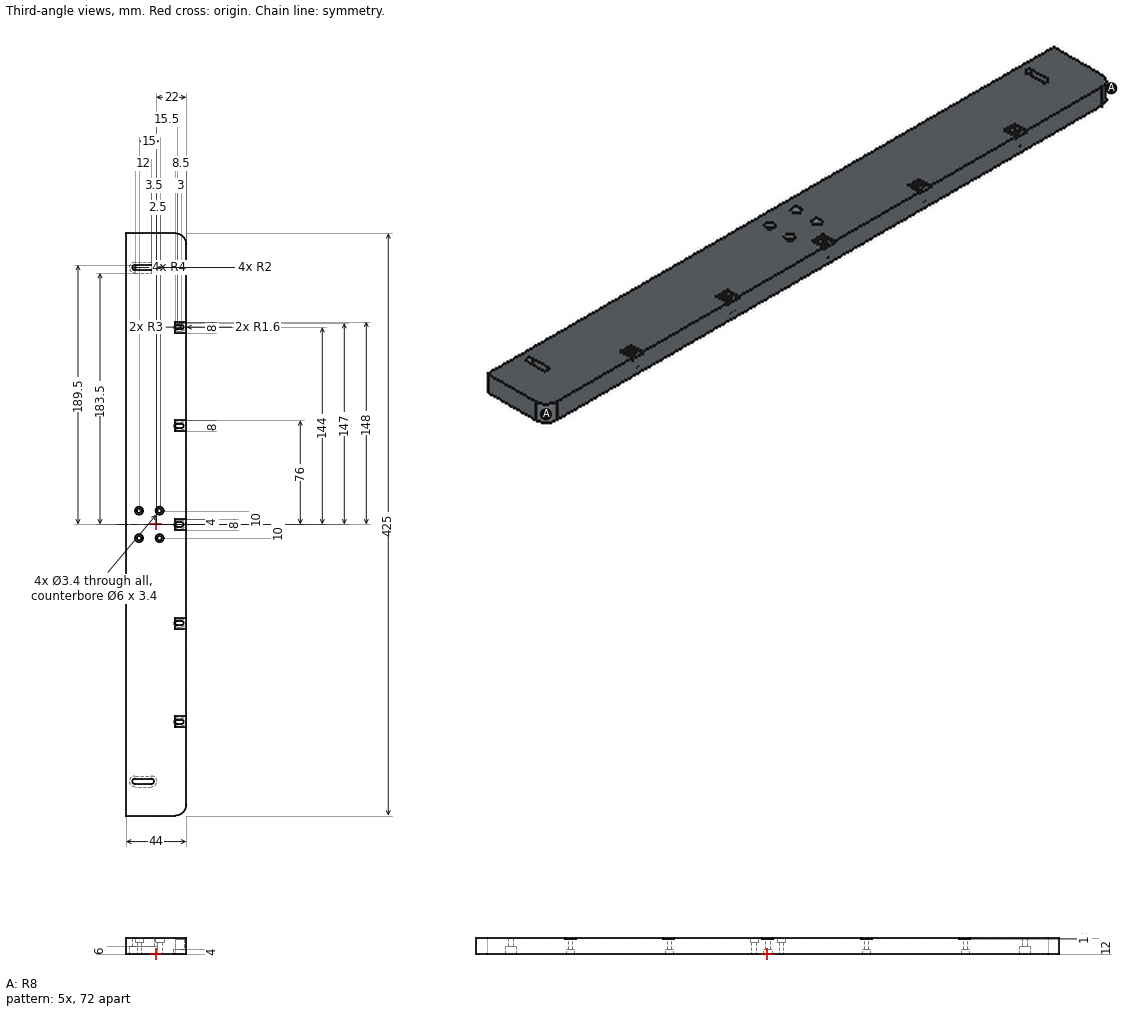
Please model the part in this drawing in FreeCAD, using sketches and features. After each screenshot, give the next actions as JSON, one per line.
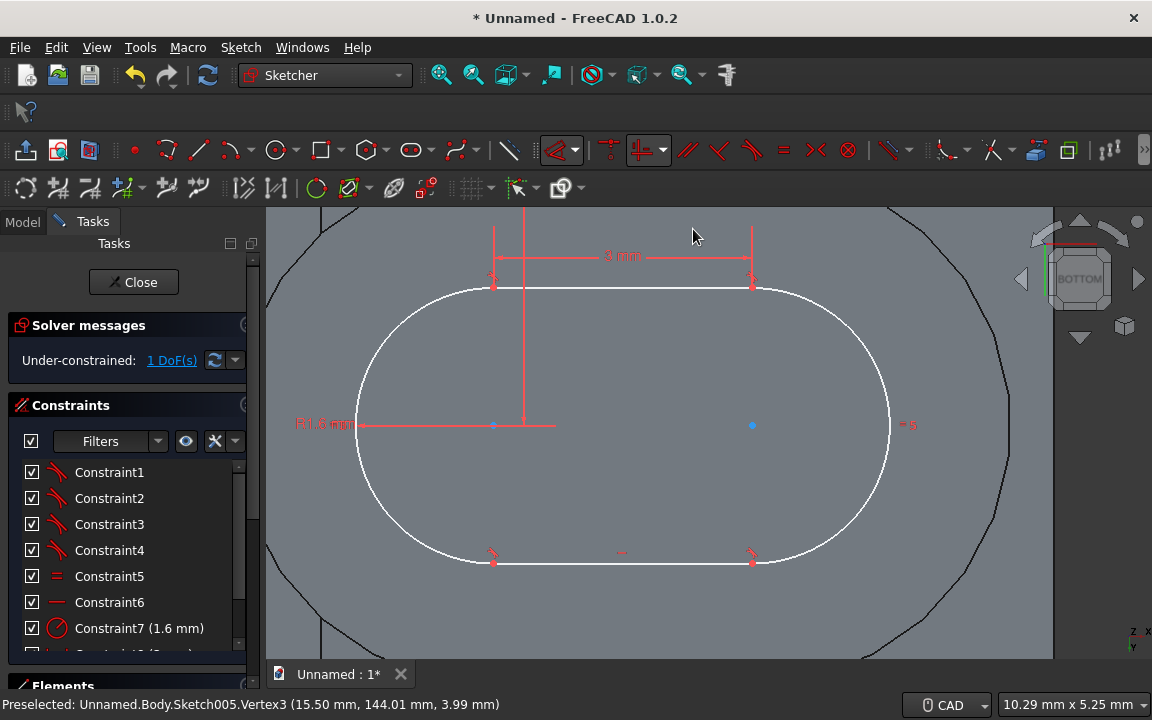
{"action": "left_click", "coordinate": [494, 288]}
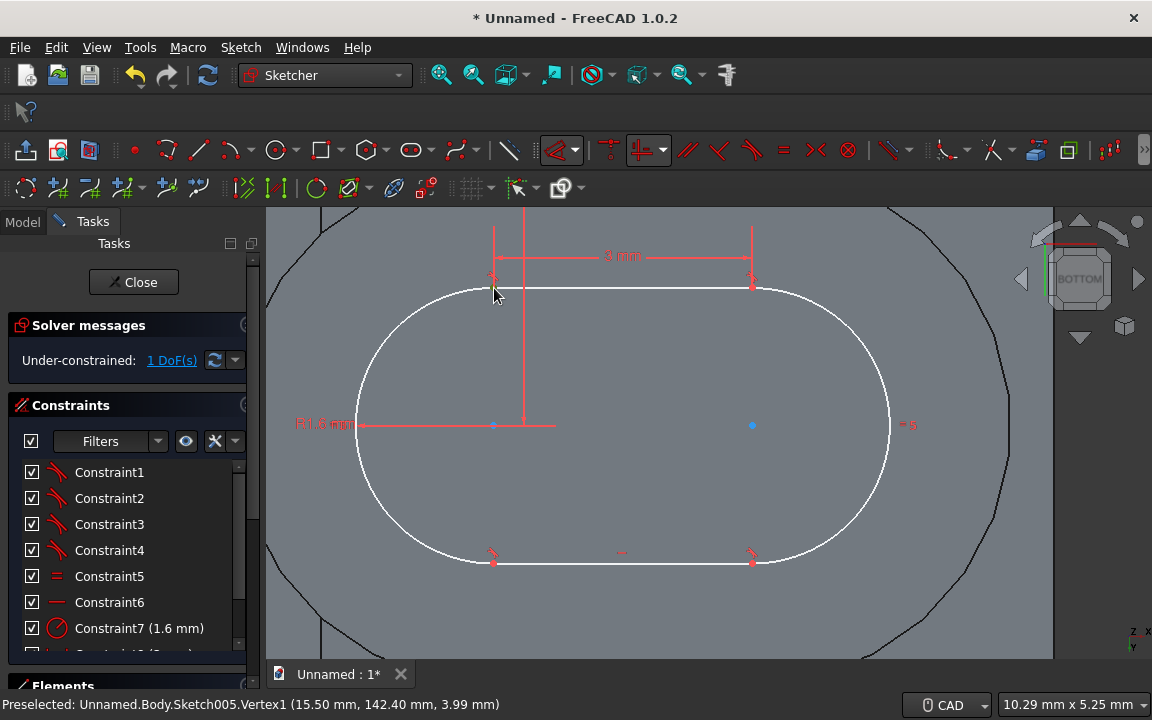
{"action": "left_click", "coordinate": [578, 150]}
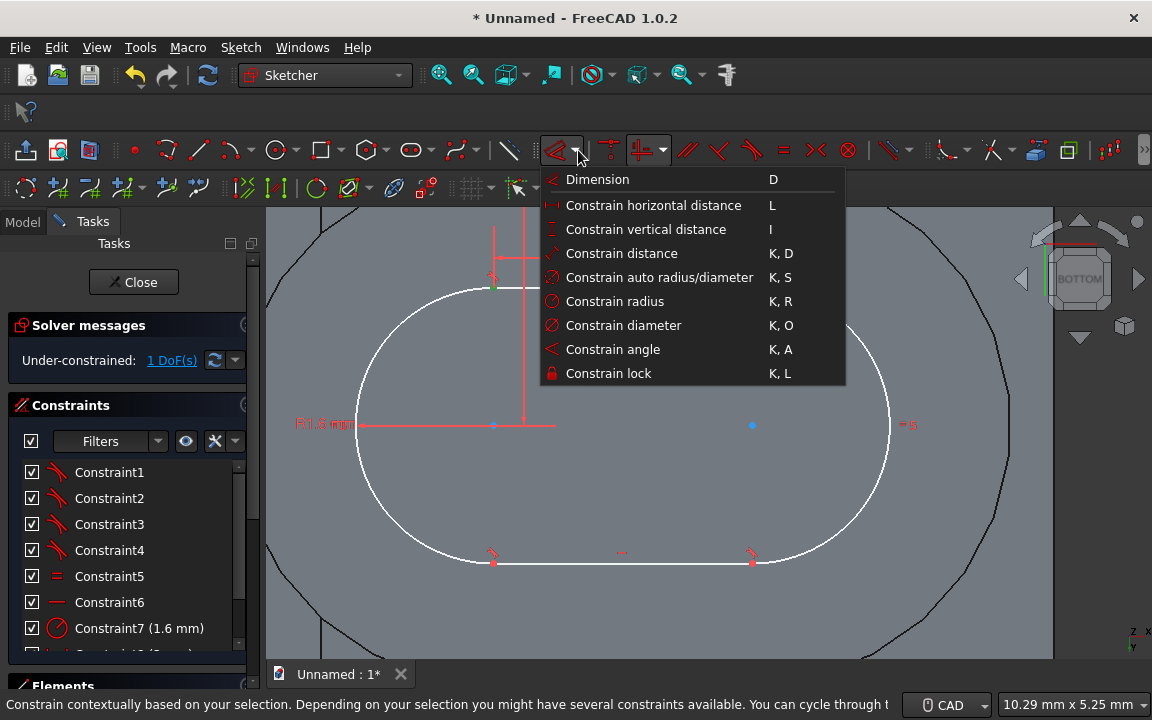
{"action": "left_click", "coordinate": [693, 205]}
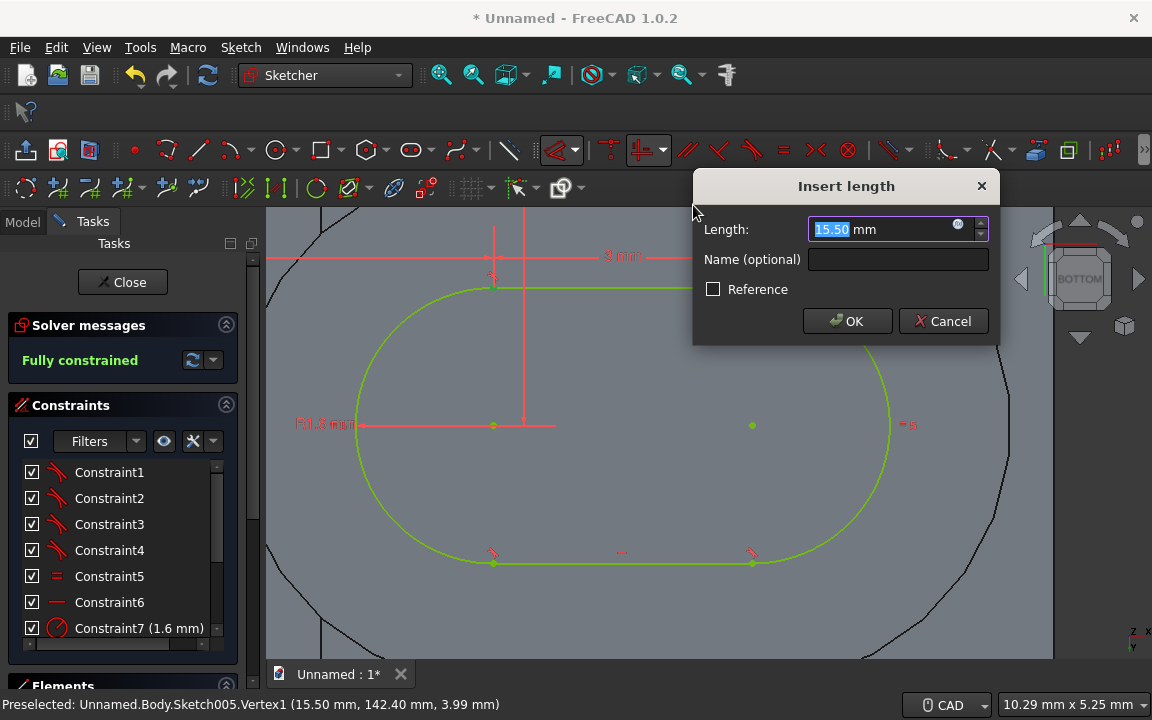
{"action": "type", "text": "15.5"}
{"action": "key", "text": "Return"}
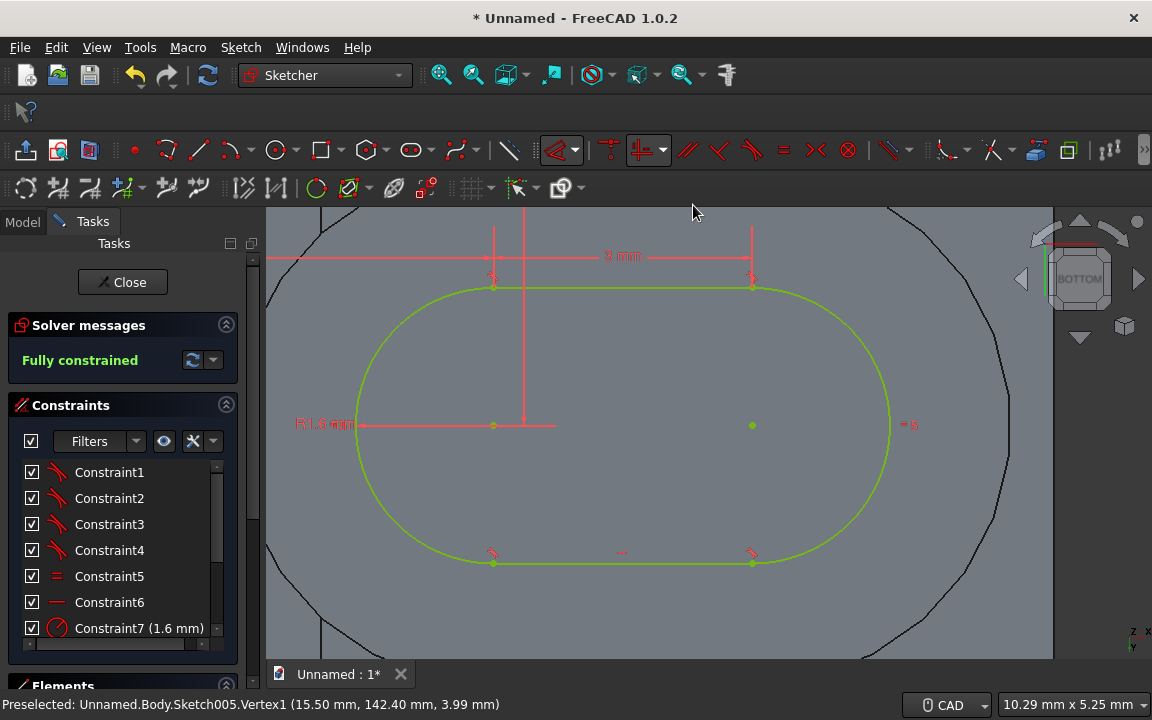
{"action": "left_click", "coordinate": [123, 282]}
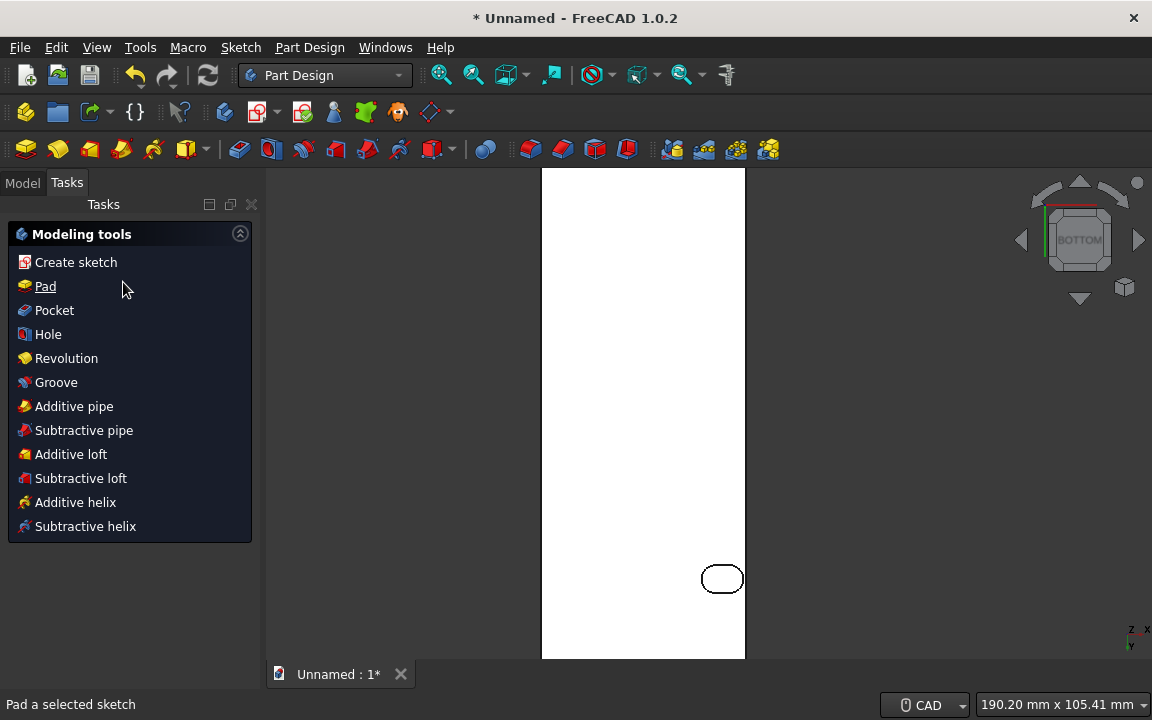
{"action": "left_click", "coordinate": [240, 150]}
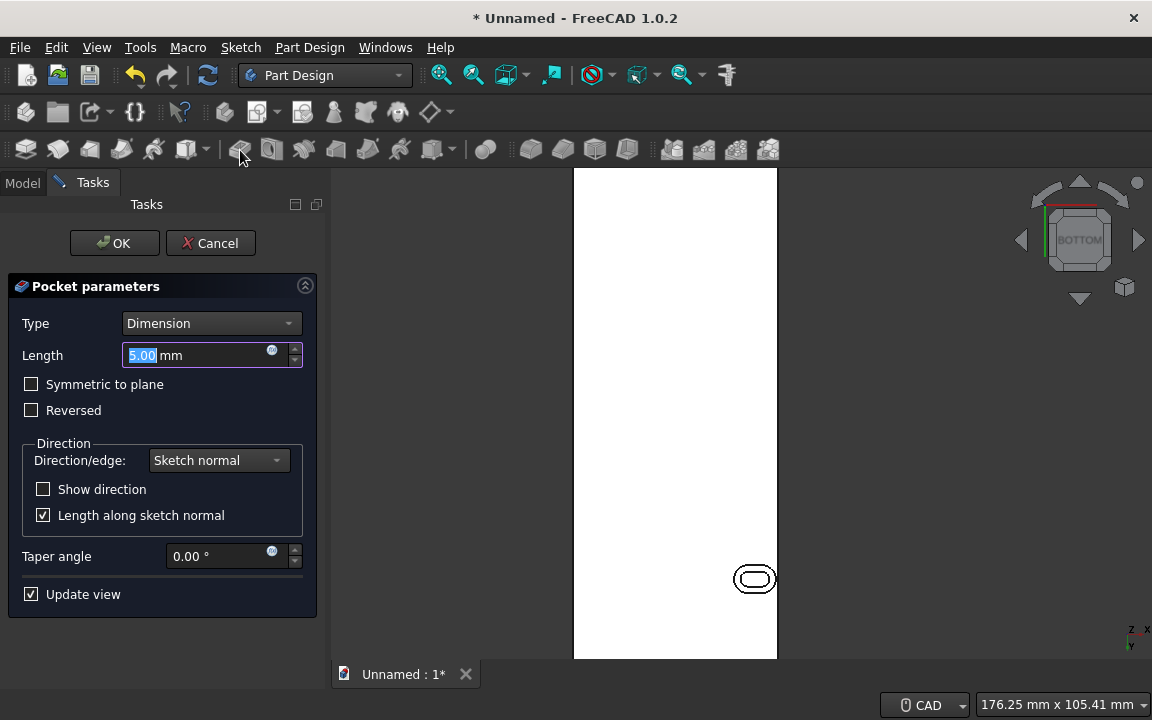
{"action": "left_click", "coordinate": [212, 324]}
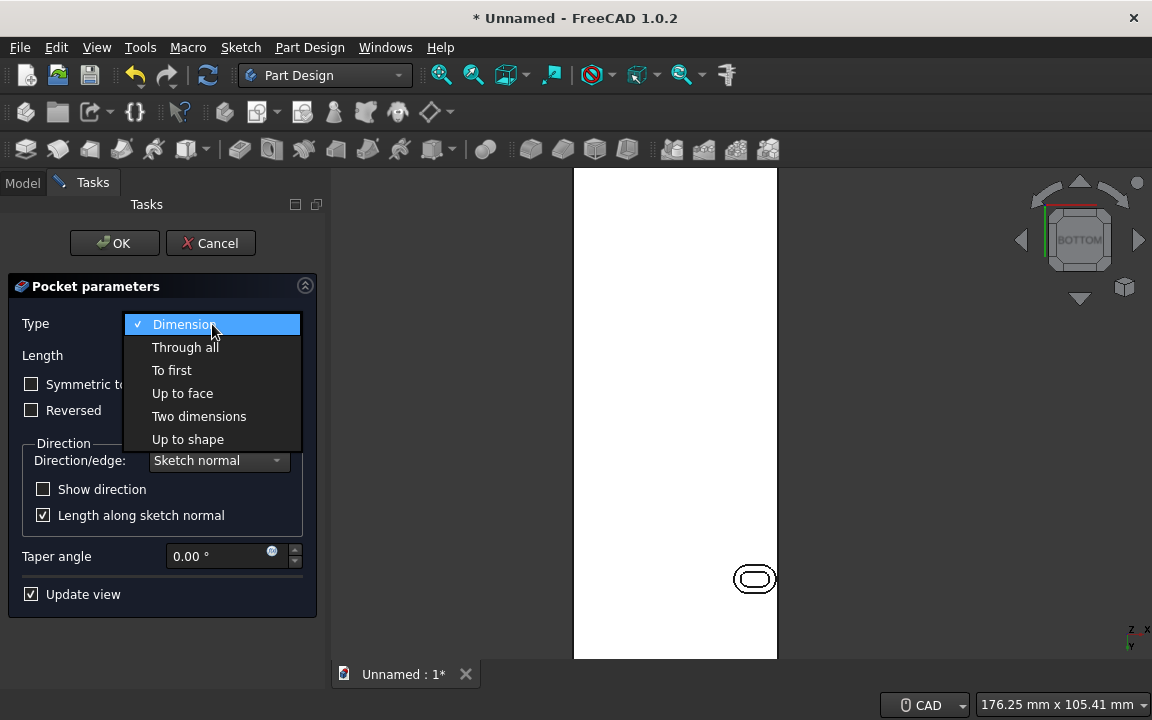
{"action": "left_click", "coordinate": [212, 348]}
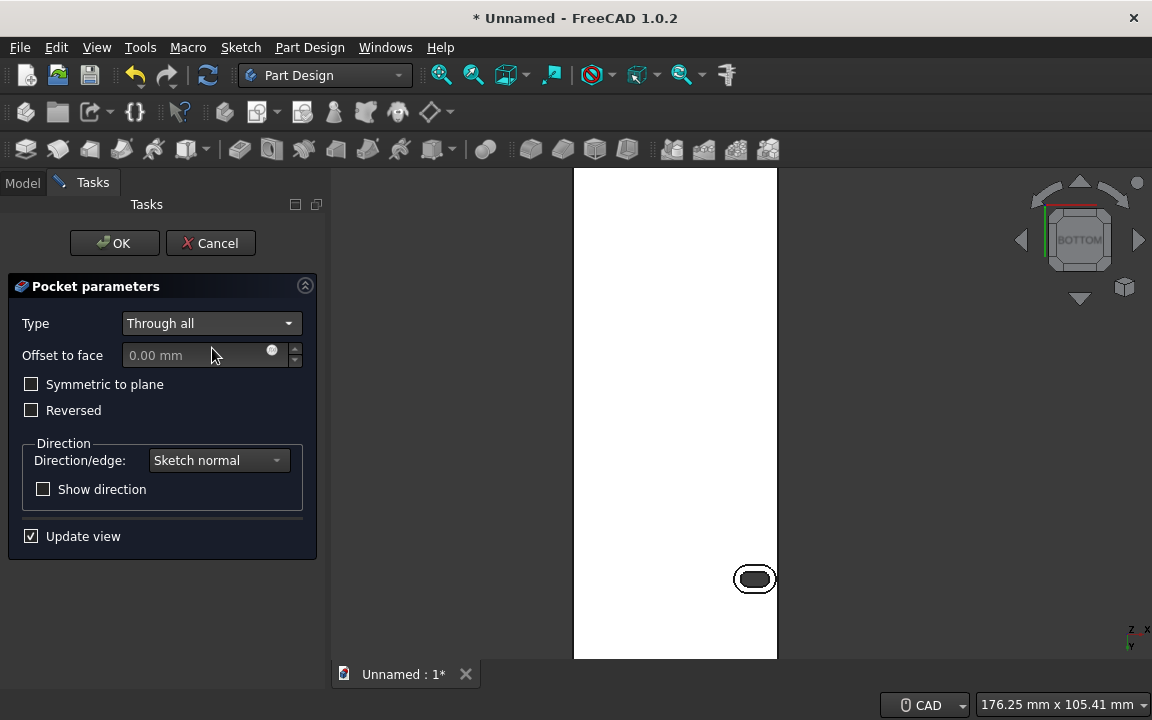
{"action": "left_click", "coordinate": [115, 243]}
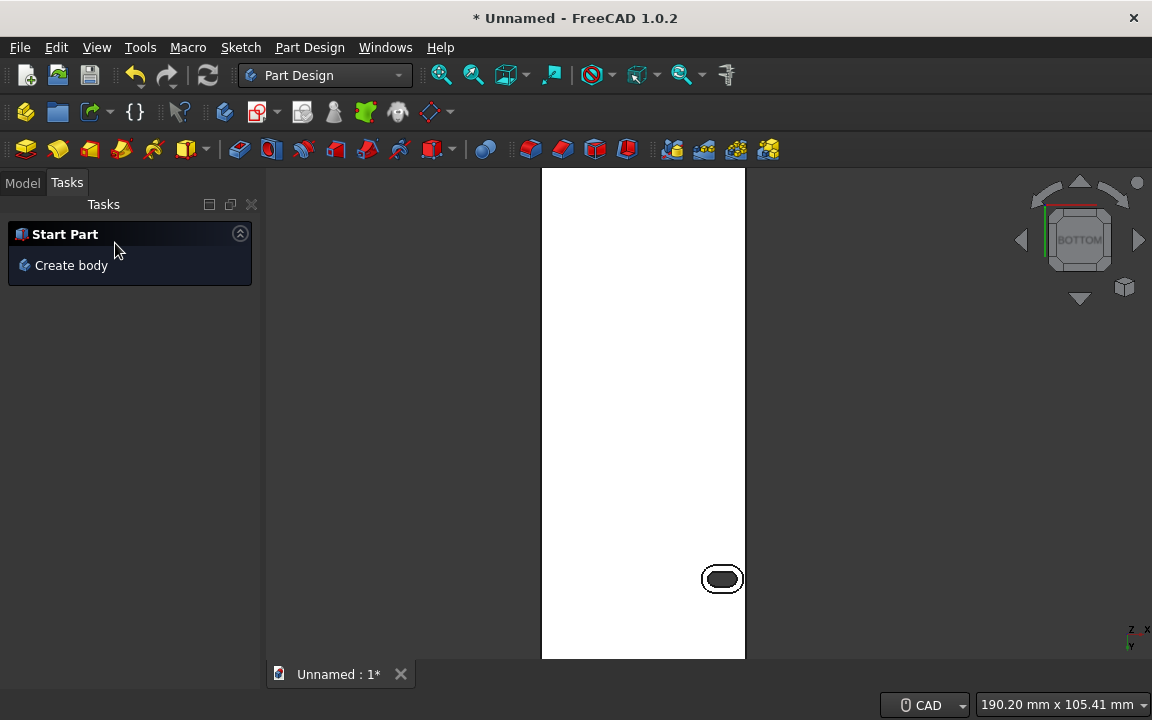
{"action": "key", "text": "v f"}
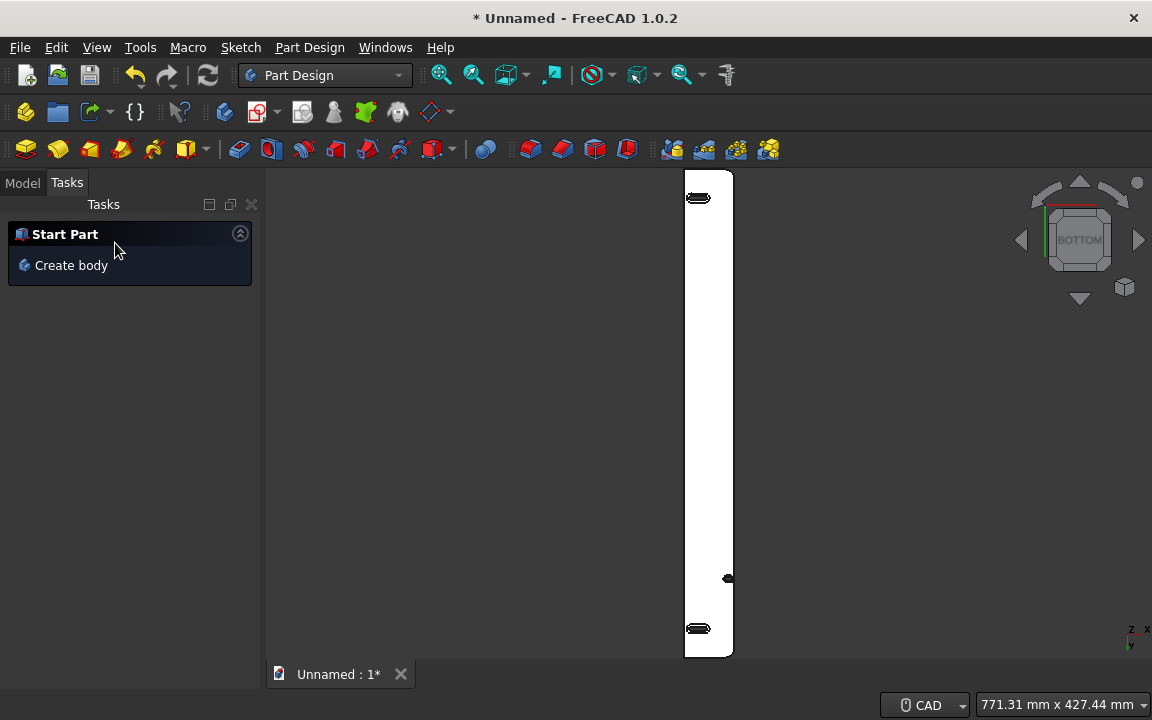
{"action": "left_click", "coordinate": [23, 182]}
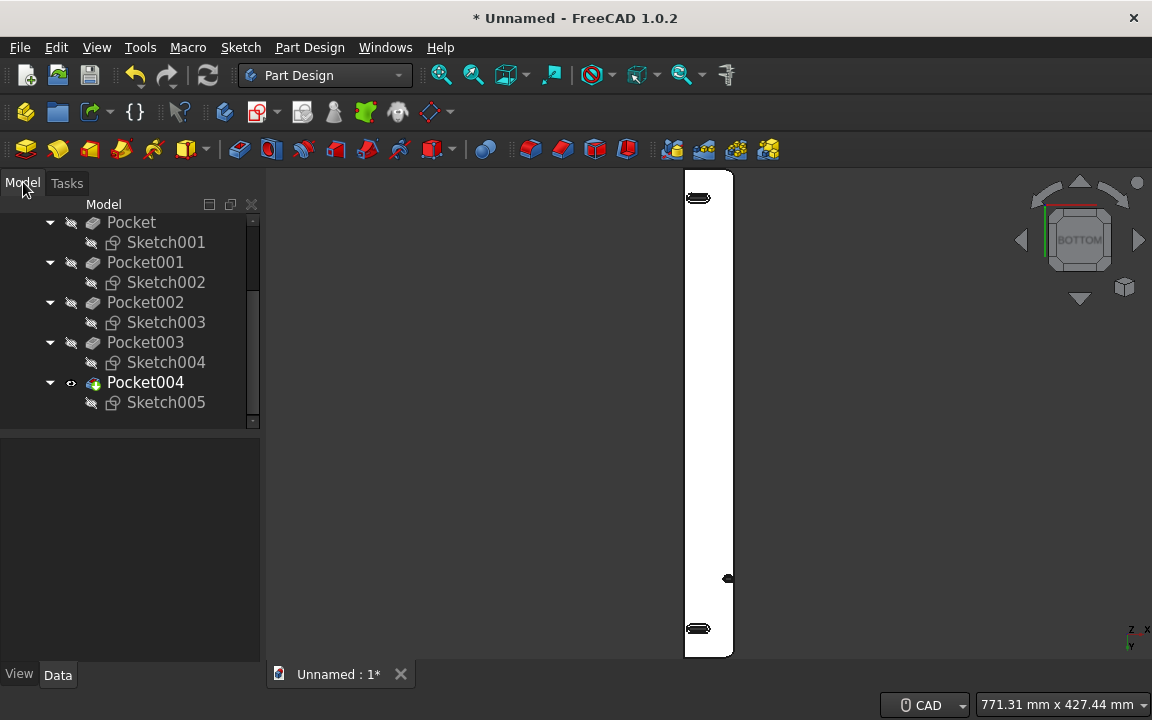
{"action": "left_click", "coordinate": [116, 343]}